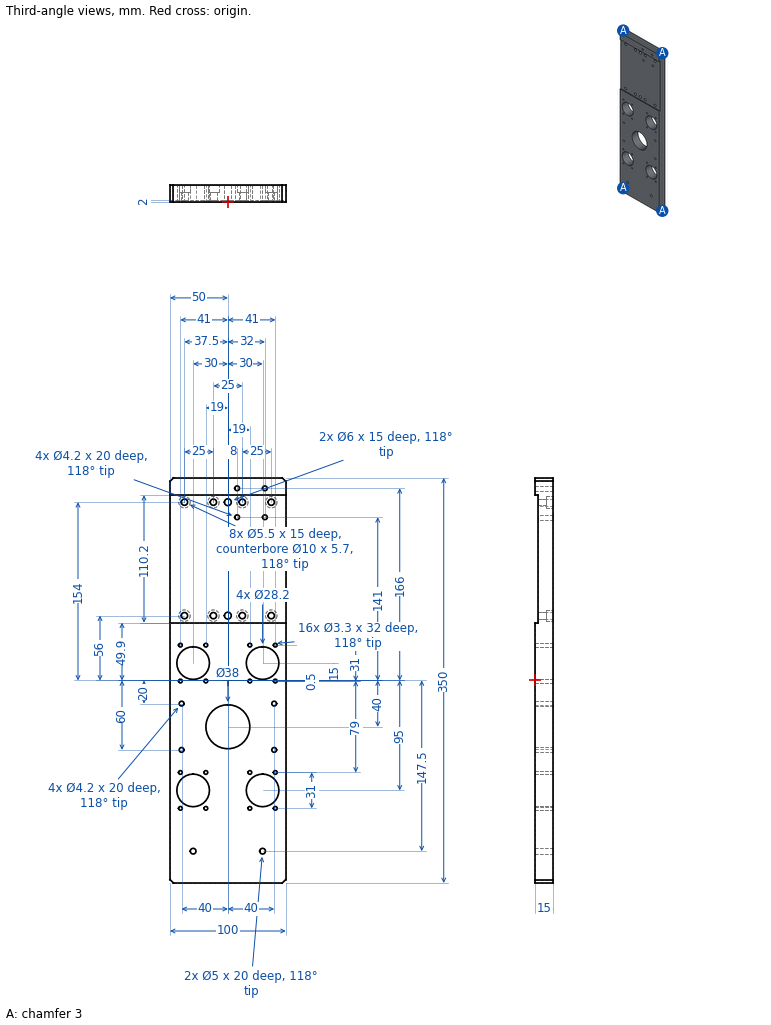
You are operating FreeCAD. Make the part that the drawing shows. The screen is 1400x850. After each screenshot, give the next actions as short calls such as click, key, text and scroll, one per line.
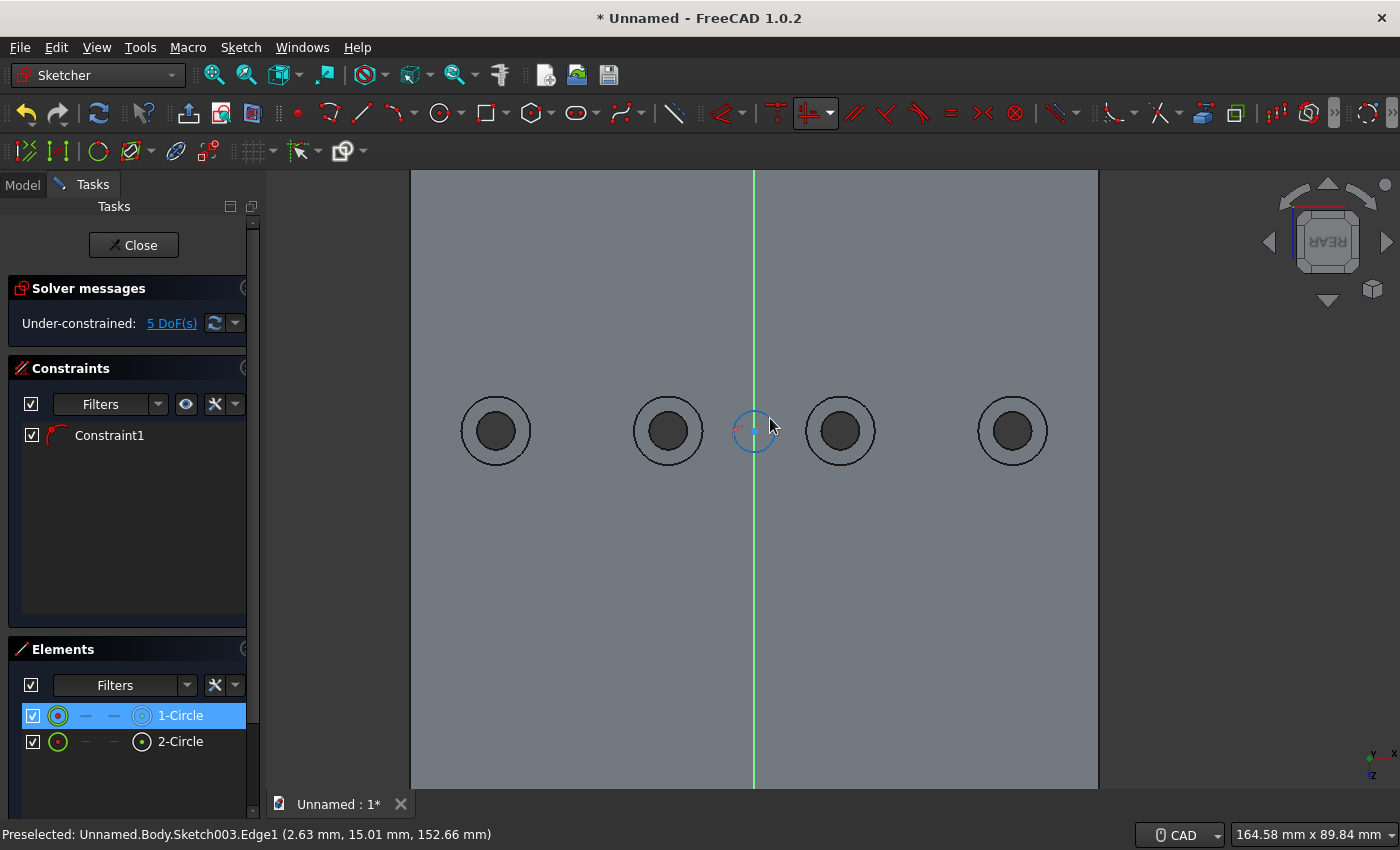
click(769, 417)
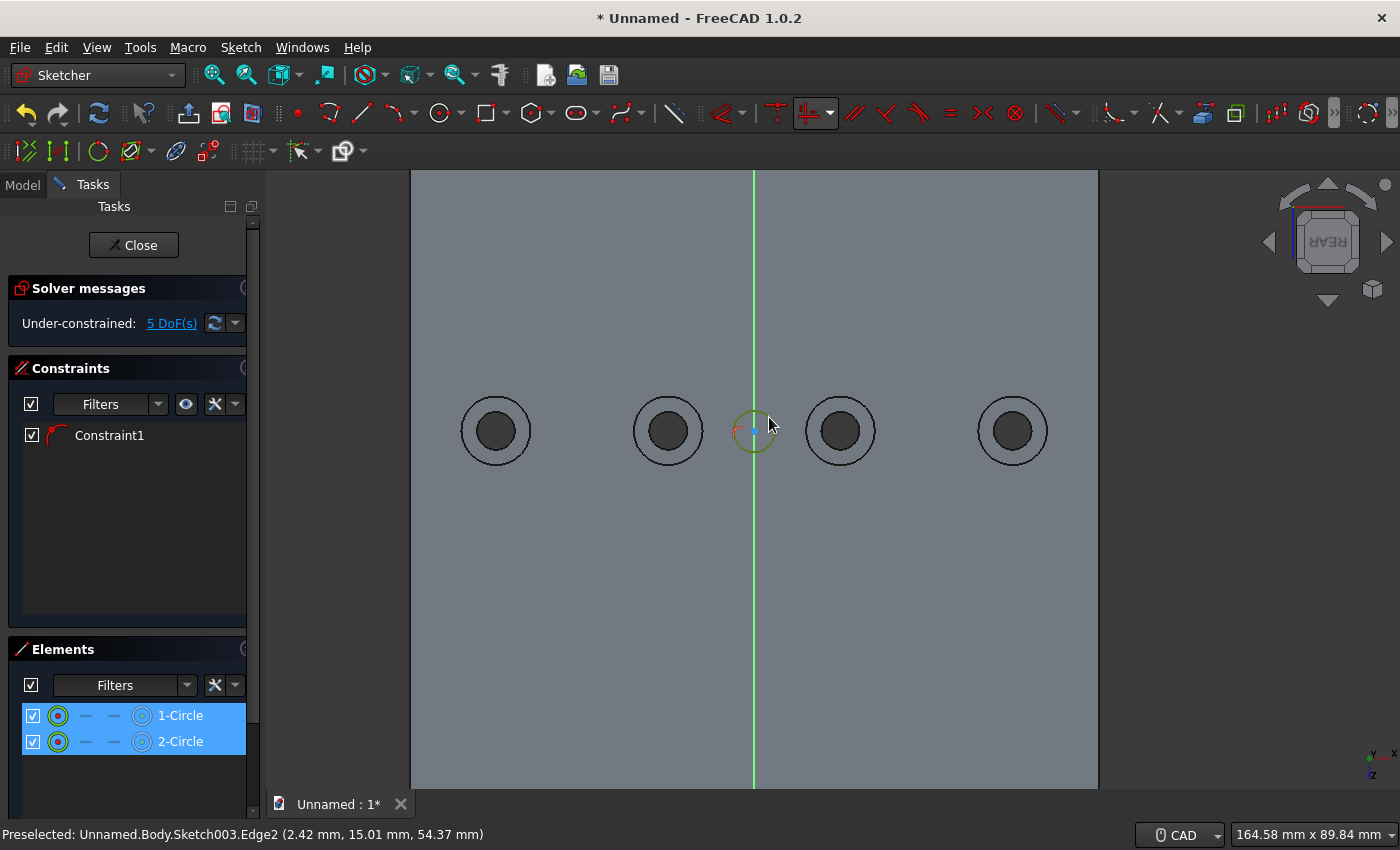
click(952, 114)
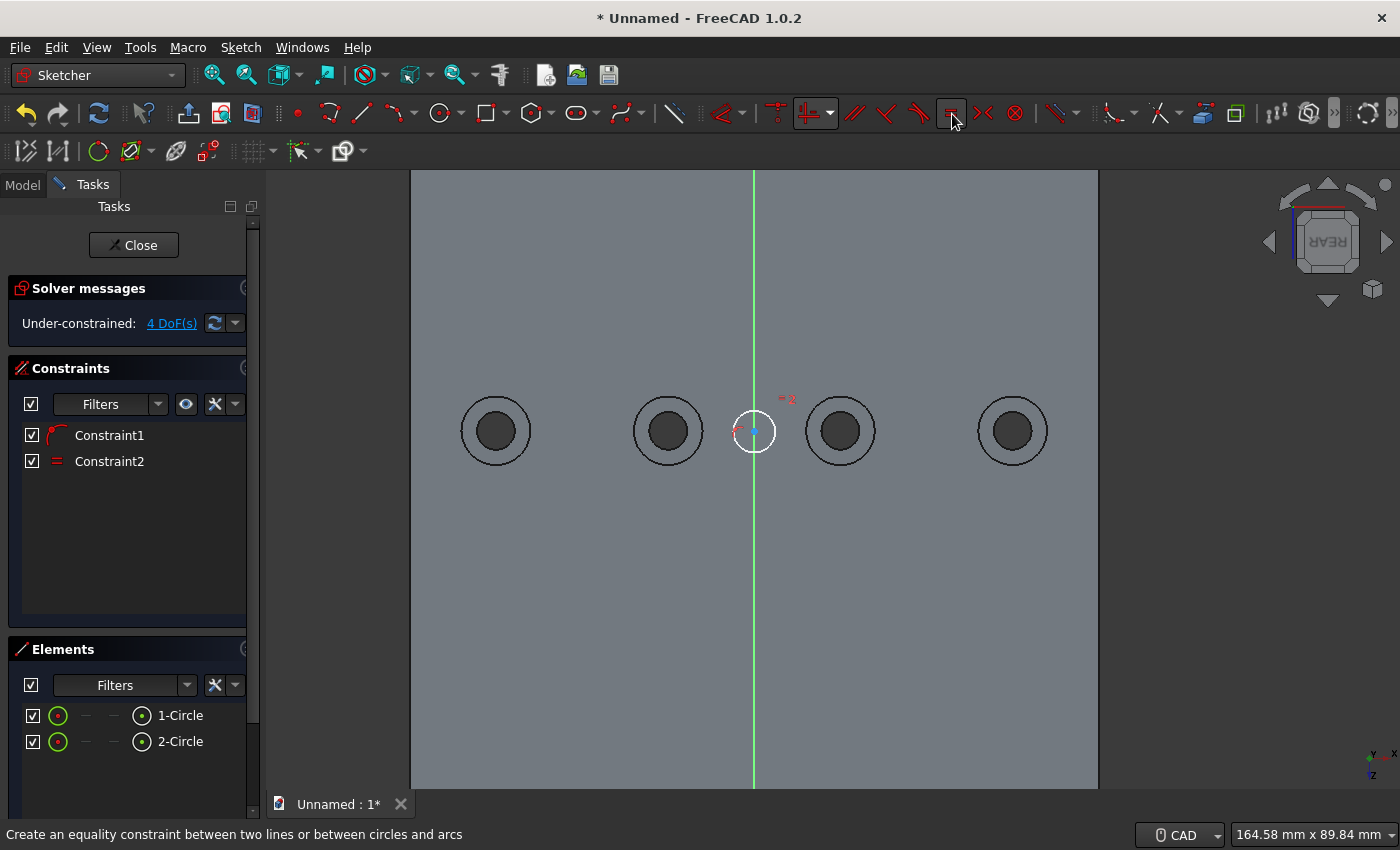
scroll(770, 418, down, 5)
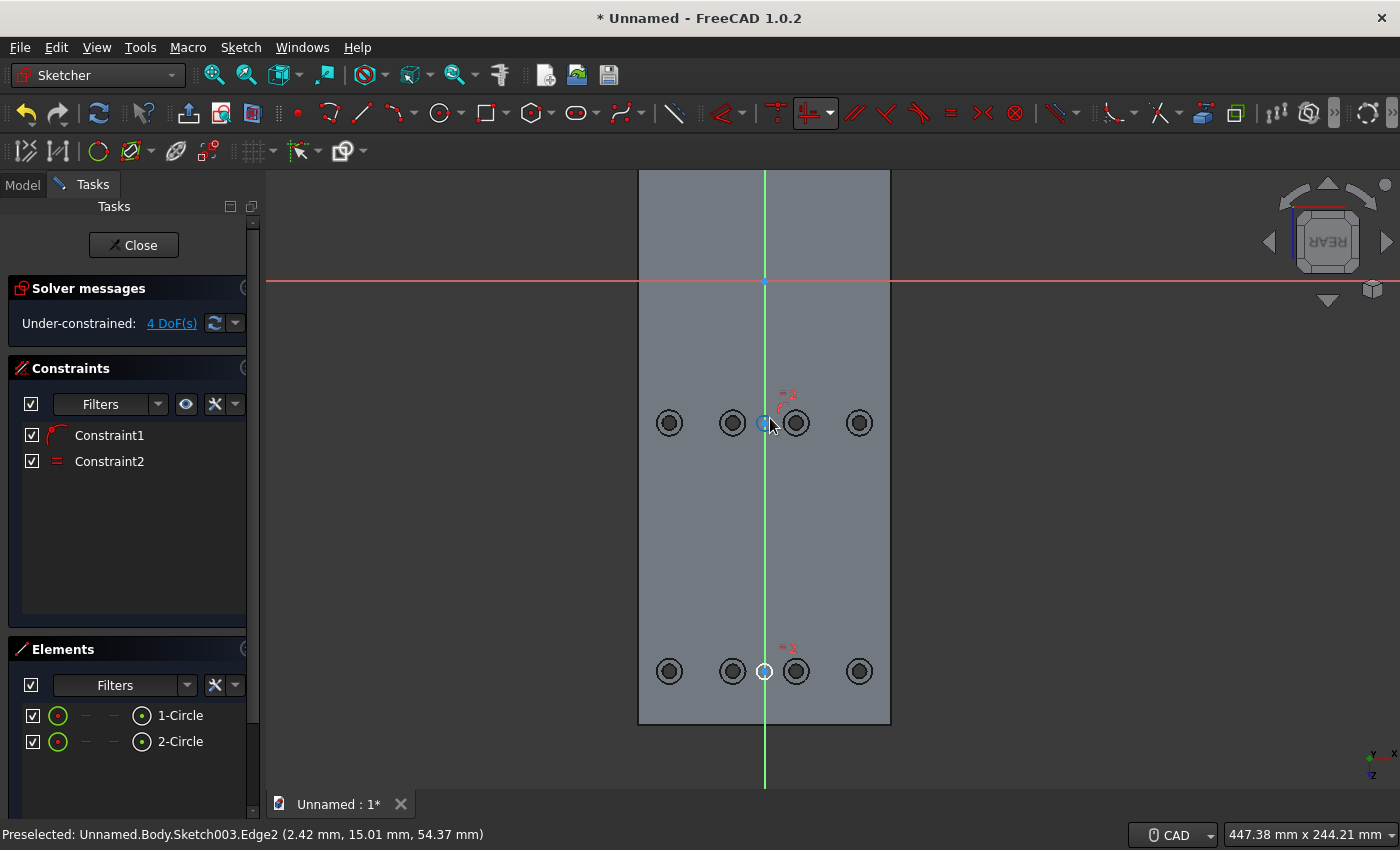
click(764, 672)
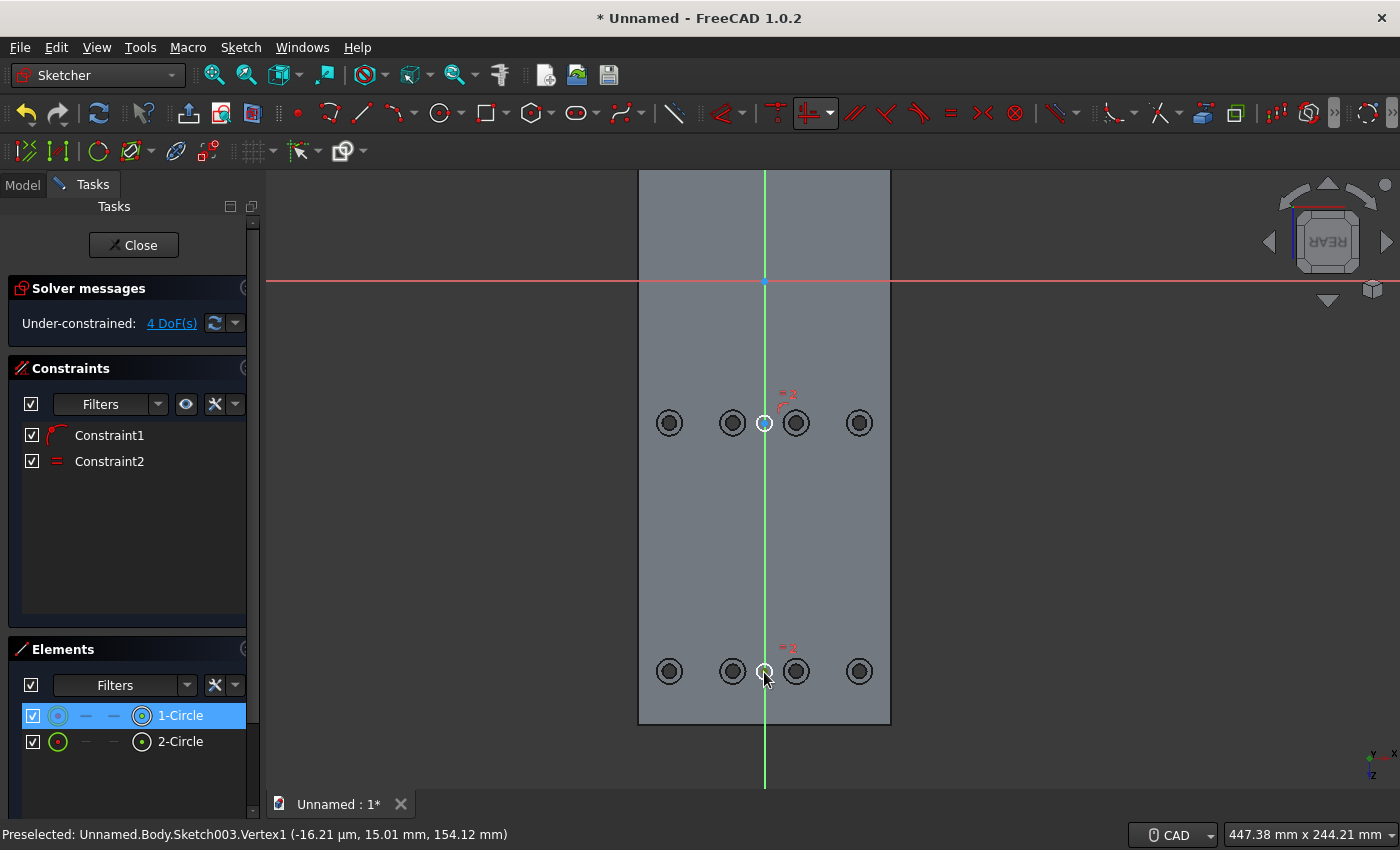
click(765, 721)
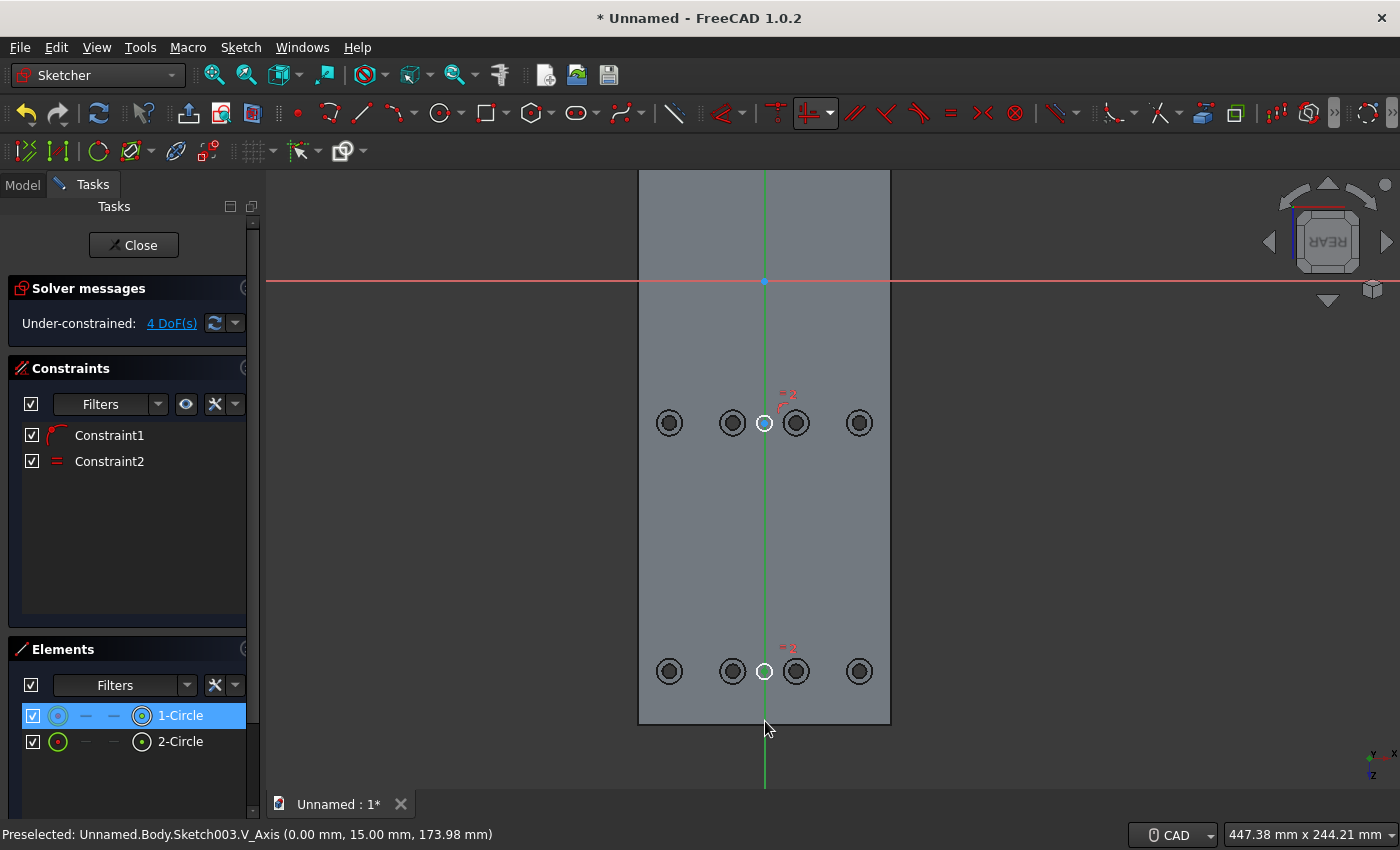
key(c)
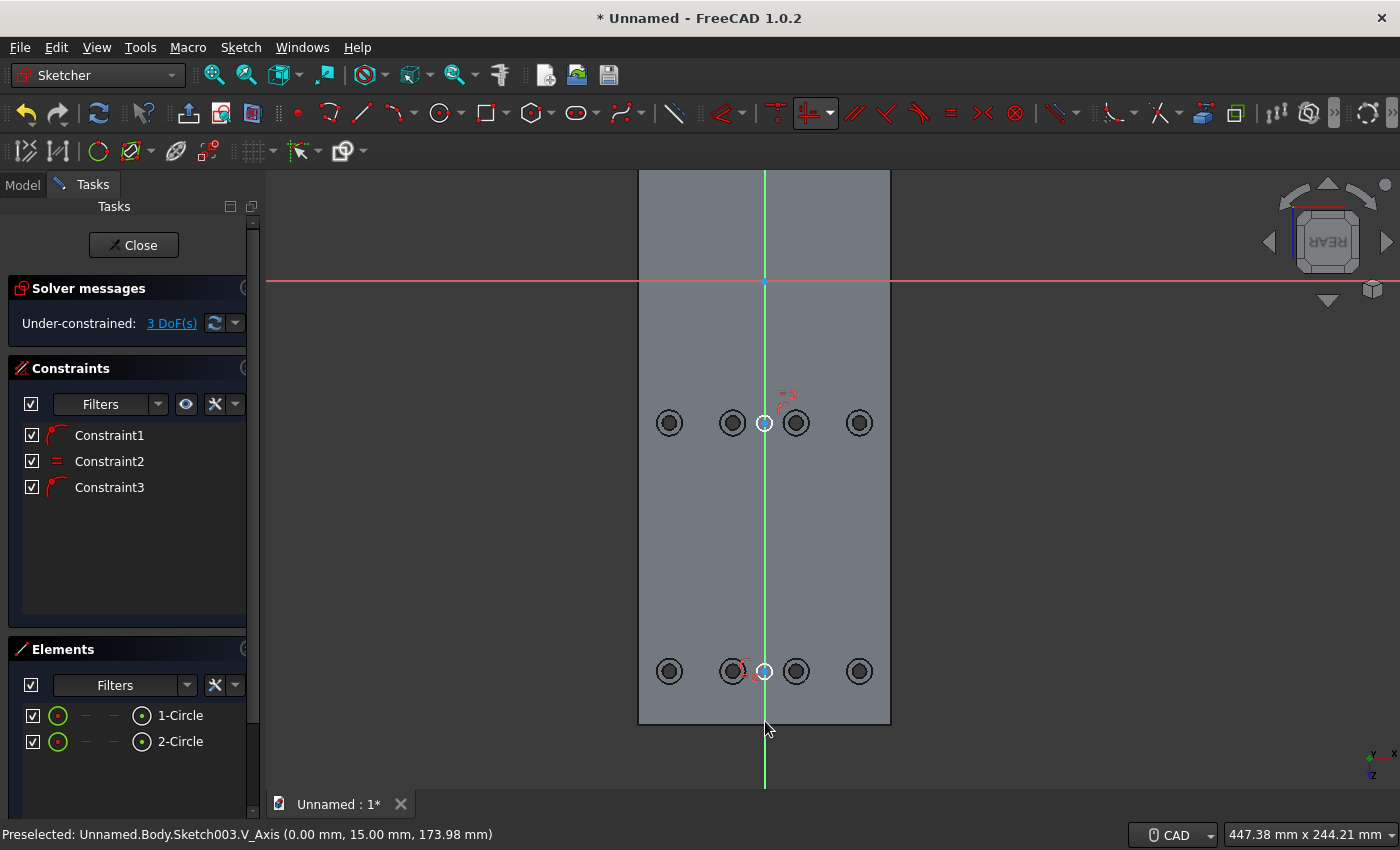
key(d)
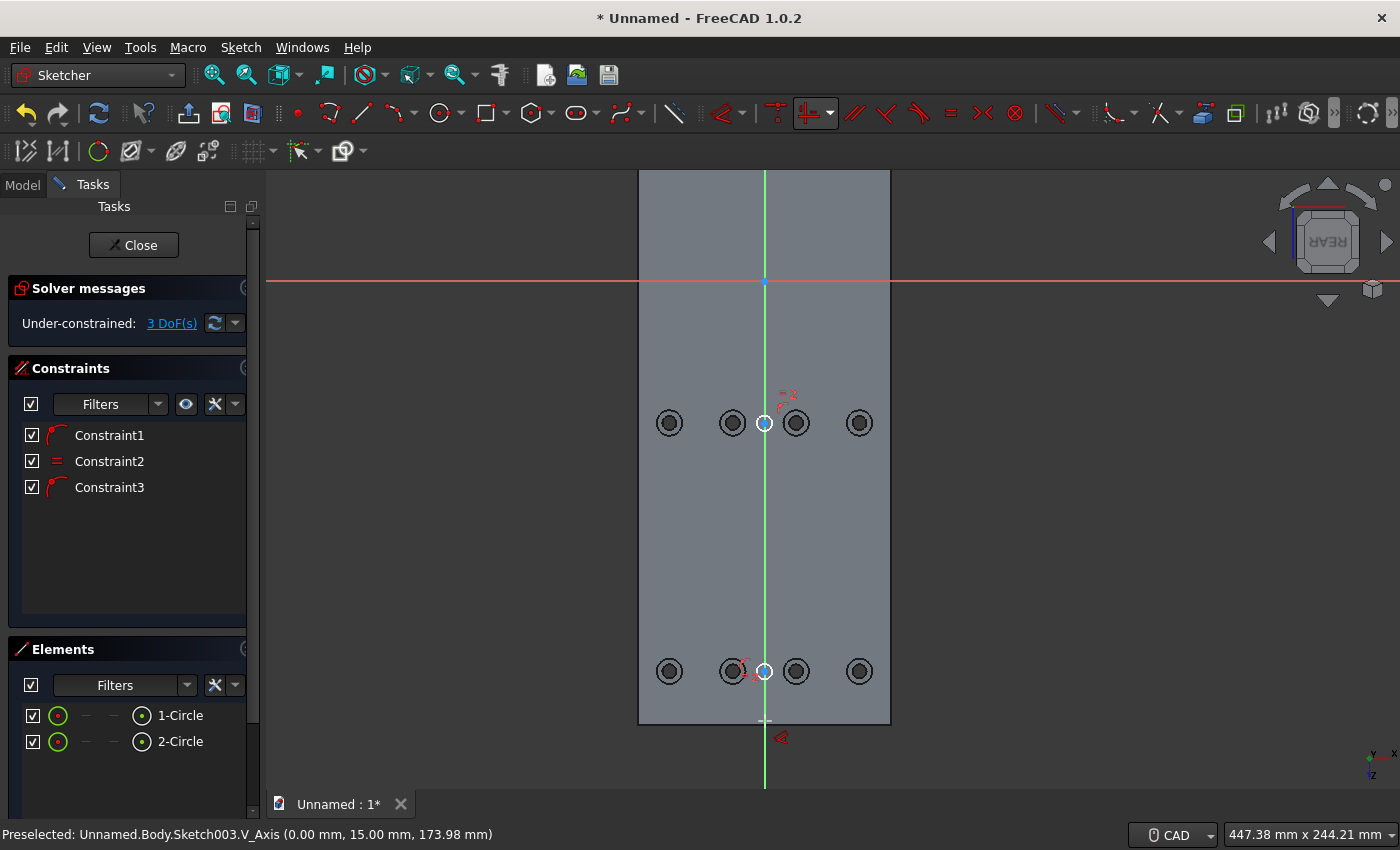
scroll(765, 664, up, 5)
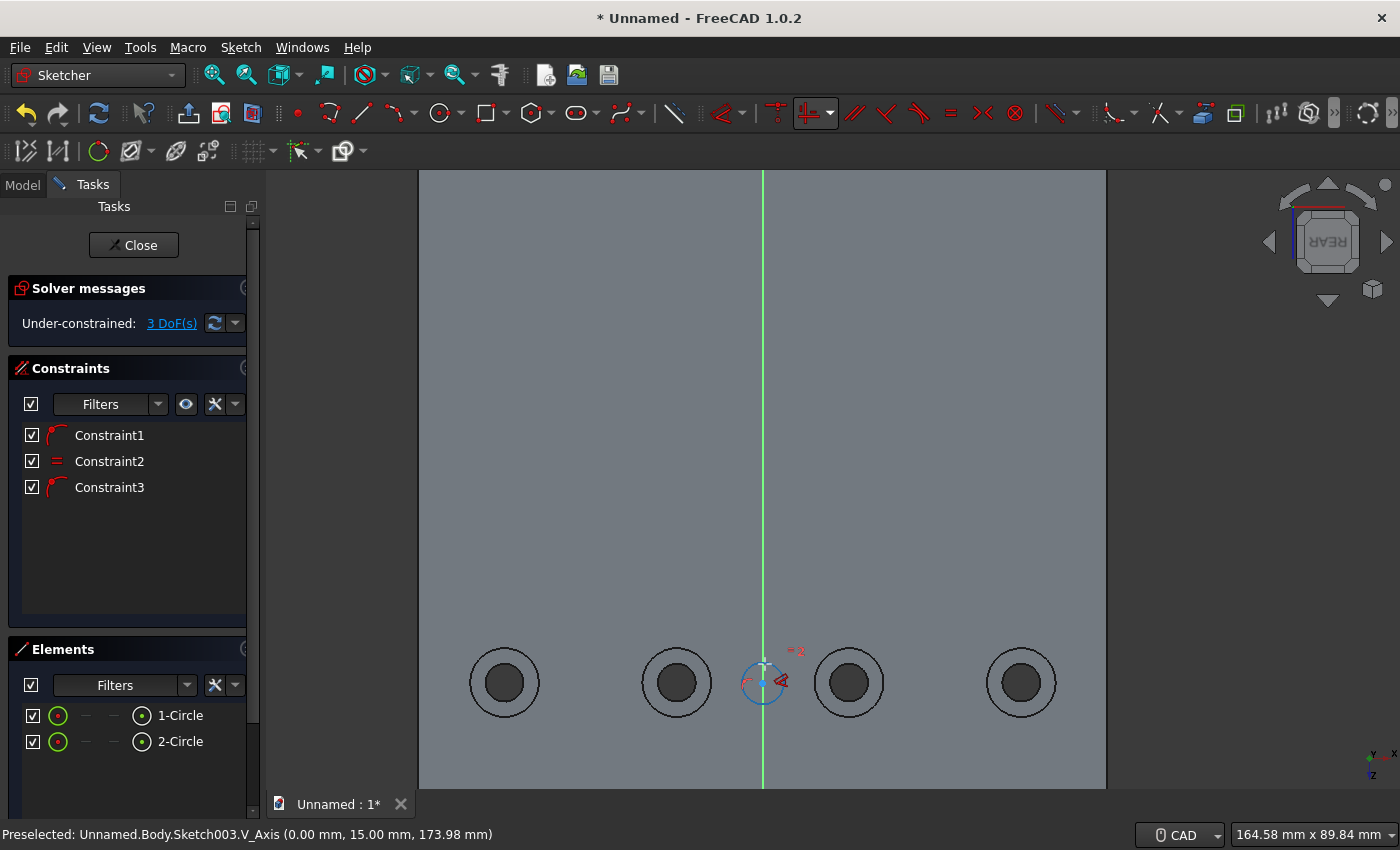
click(764, 663)
click(790, 639)